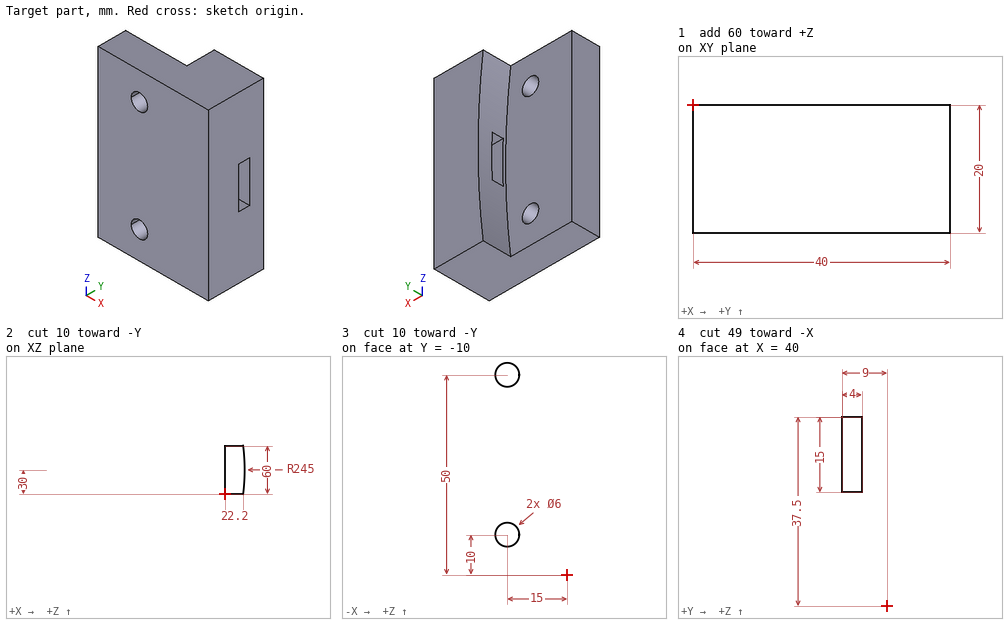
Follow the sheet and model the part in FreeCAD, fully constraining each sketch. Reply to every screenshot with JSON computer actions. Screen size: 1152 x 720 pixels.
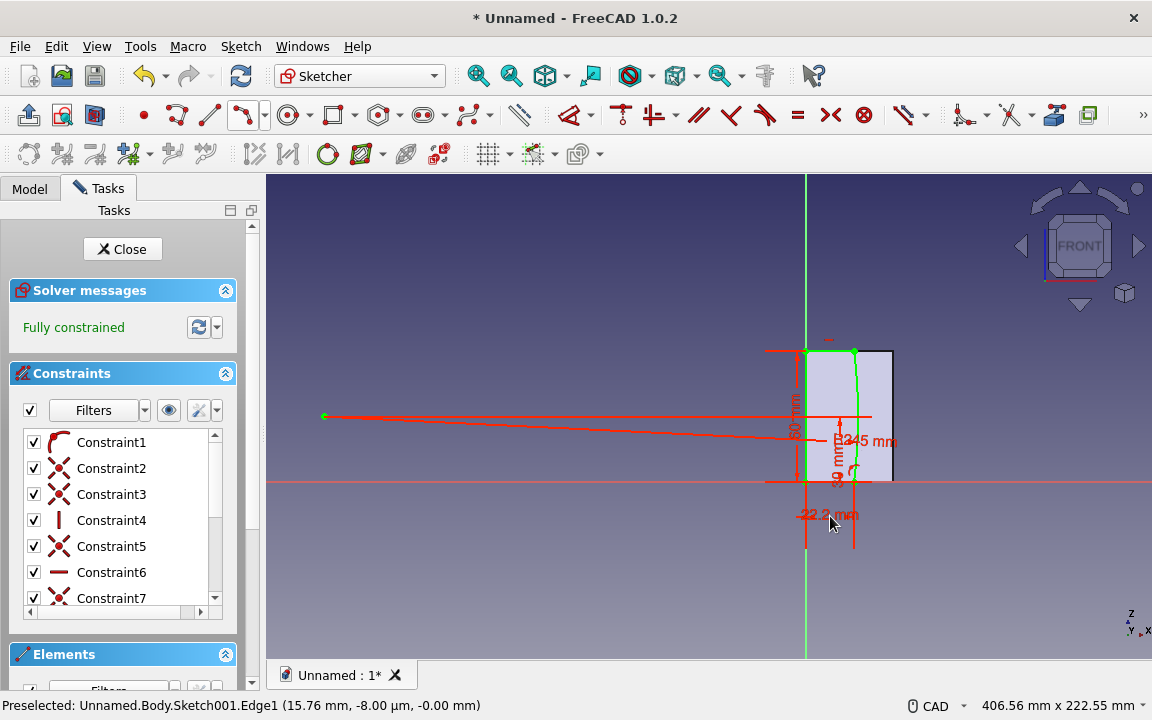
{"action": "left_click", "coordinate": [123, 249]}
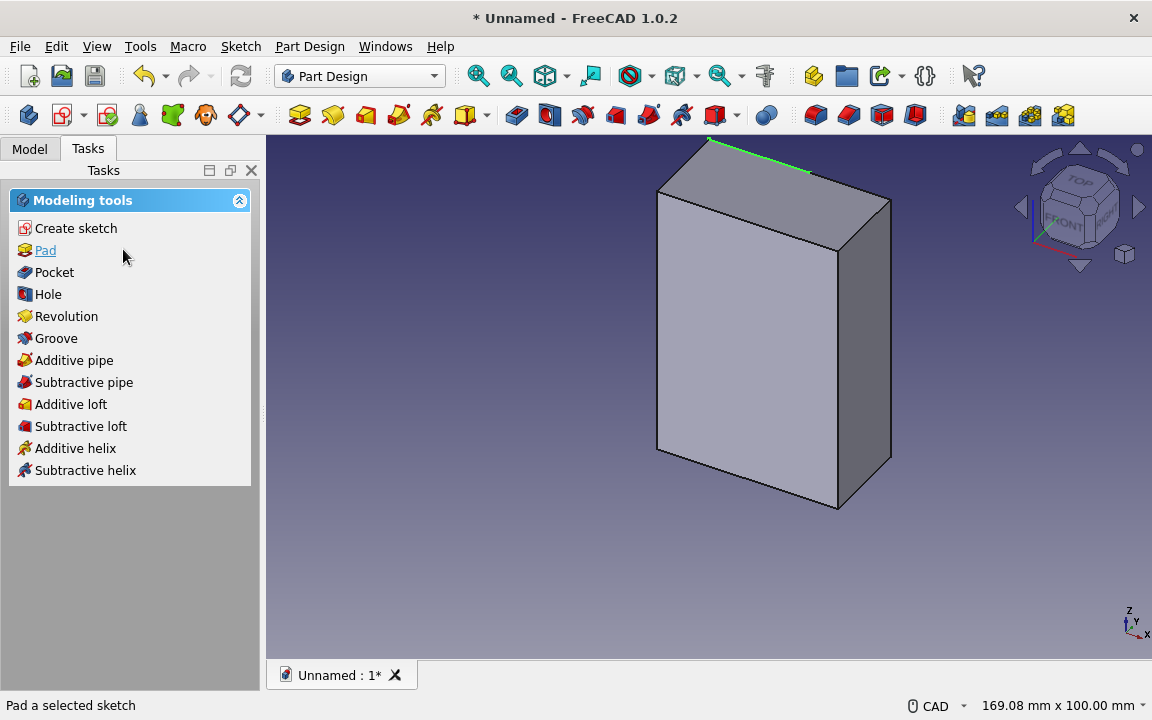
{"action": "left_click", "coordinate": [517, 116]}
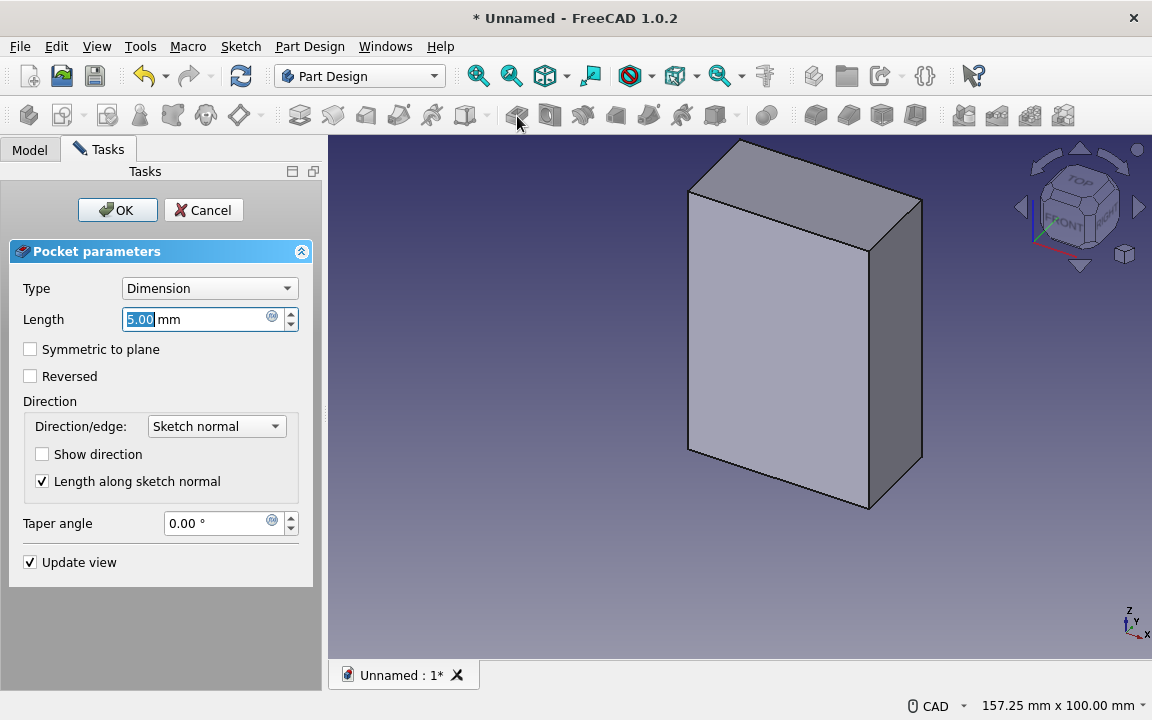
{"action": "type", "text": "10"}
{"action": "key", "text": "Tab"}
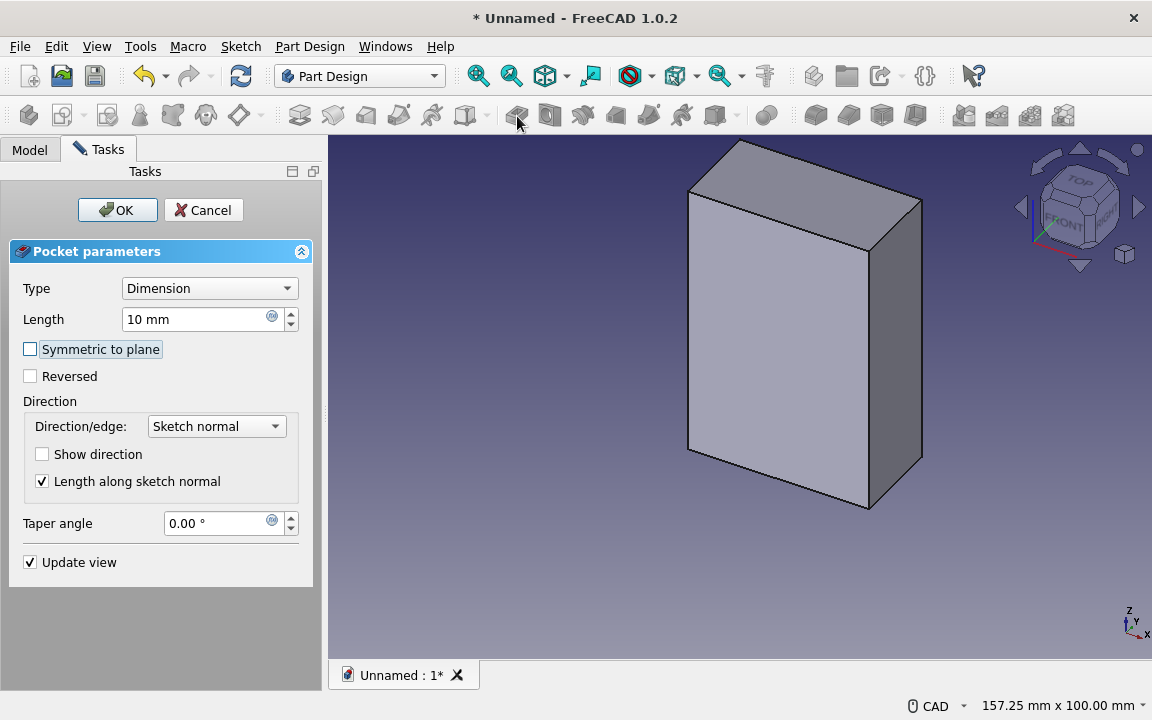
{"action": "left_click", "coordinate": [31, 376]}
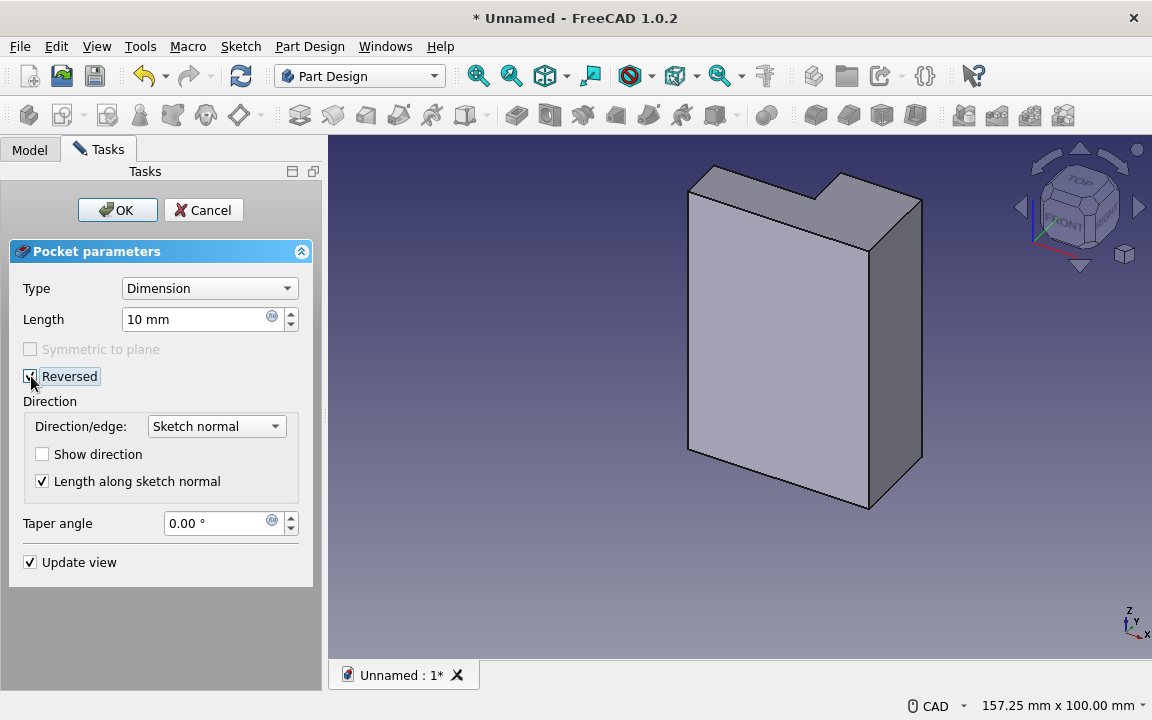
{"action": "left_click", "coordinate": [118, 210]}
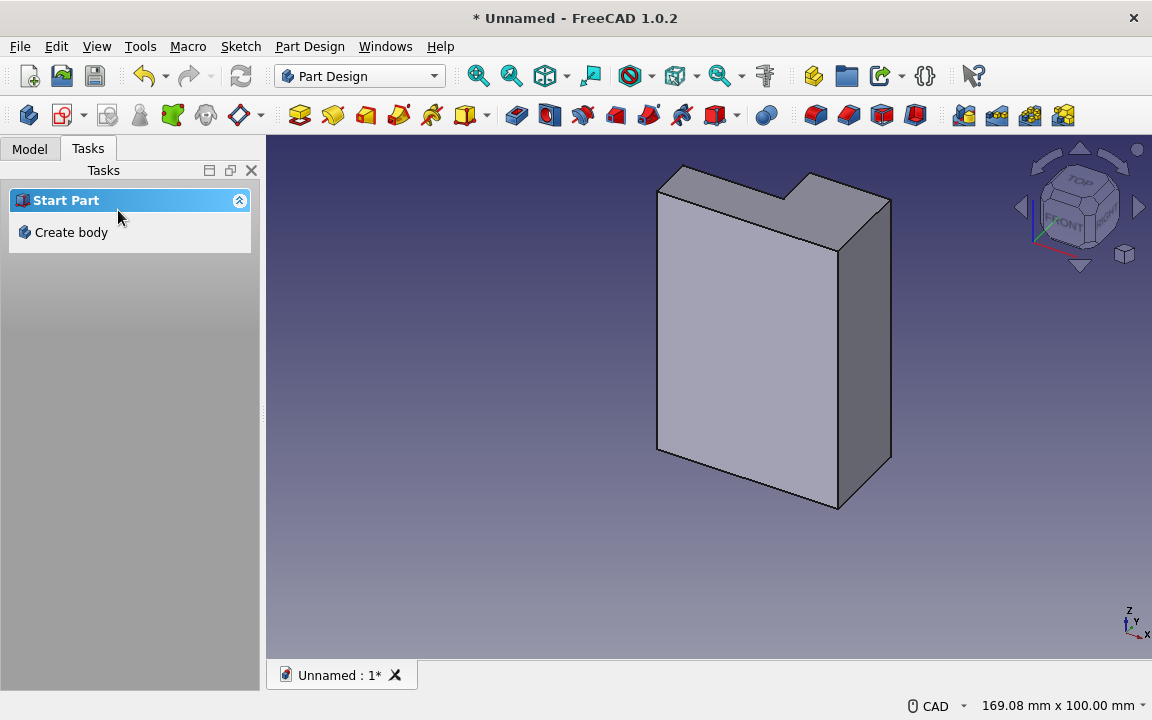
{"action": "key", "text": "4"}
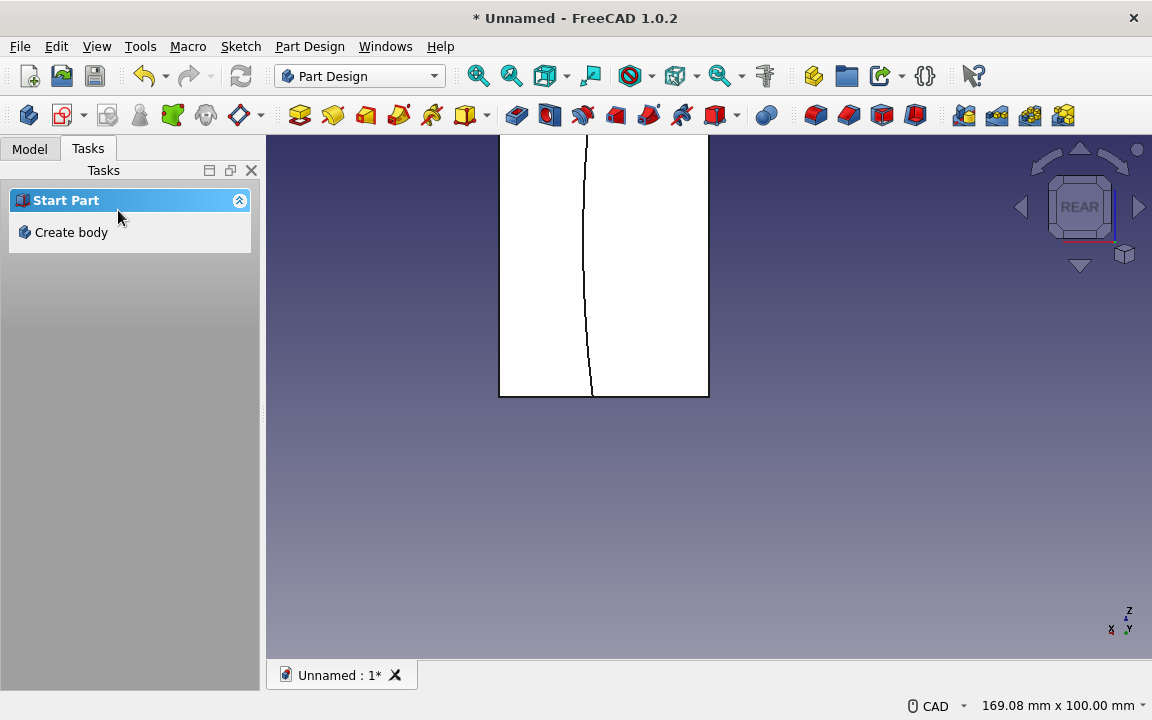
{"action": "left_click", "coordinate": [479, 76]}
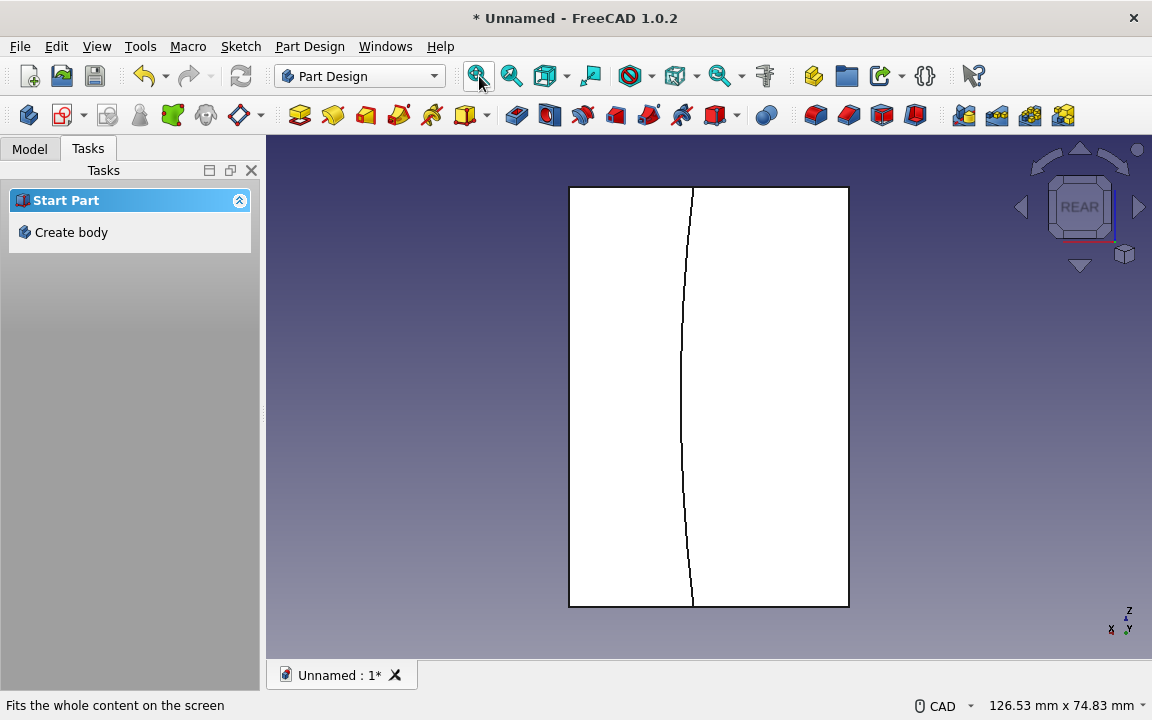
{"action": "left_click", "coordinate": [765, 396]}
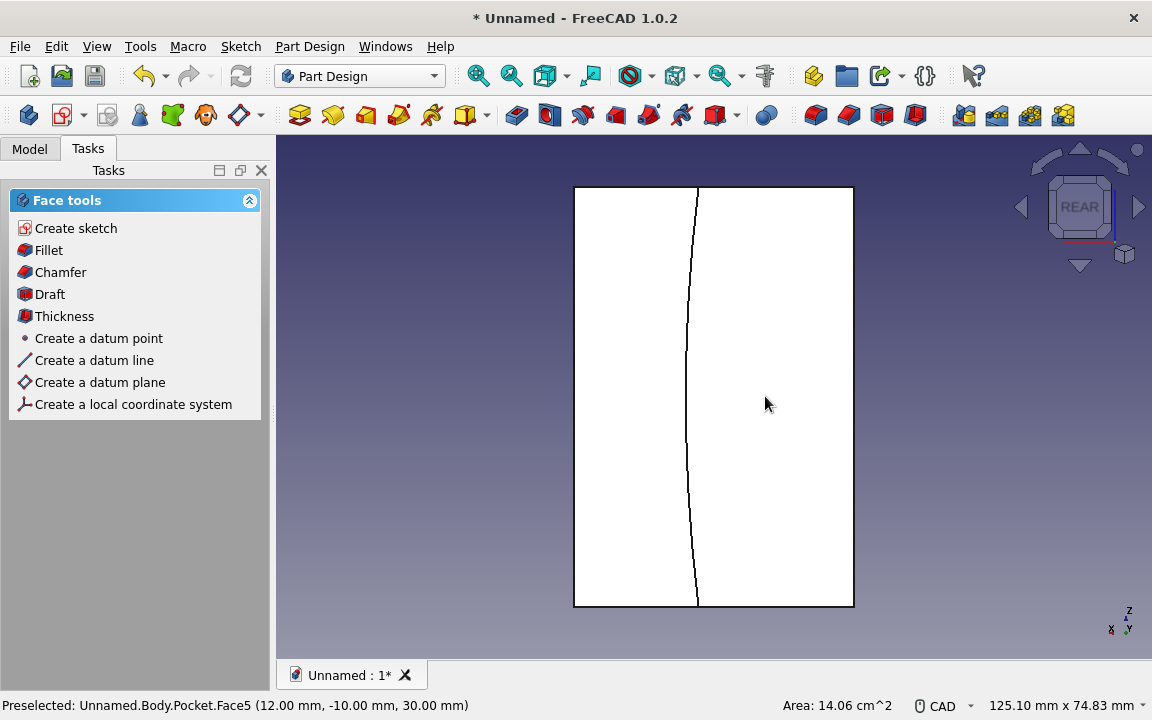
{"action": "left_click", "coordinate": [62, 116]}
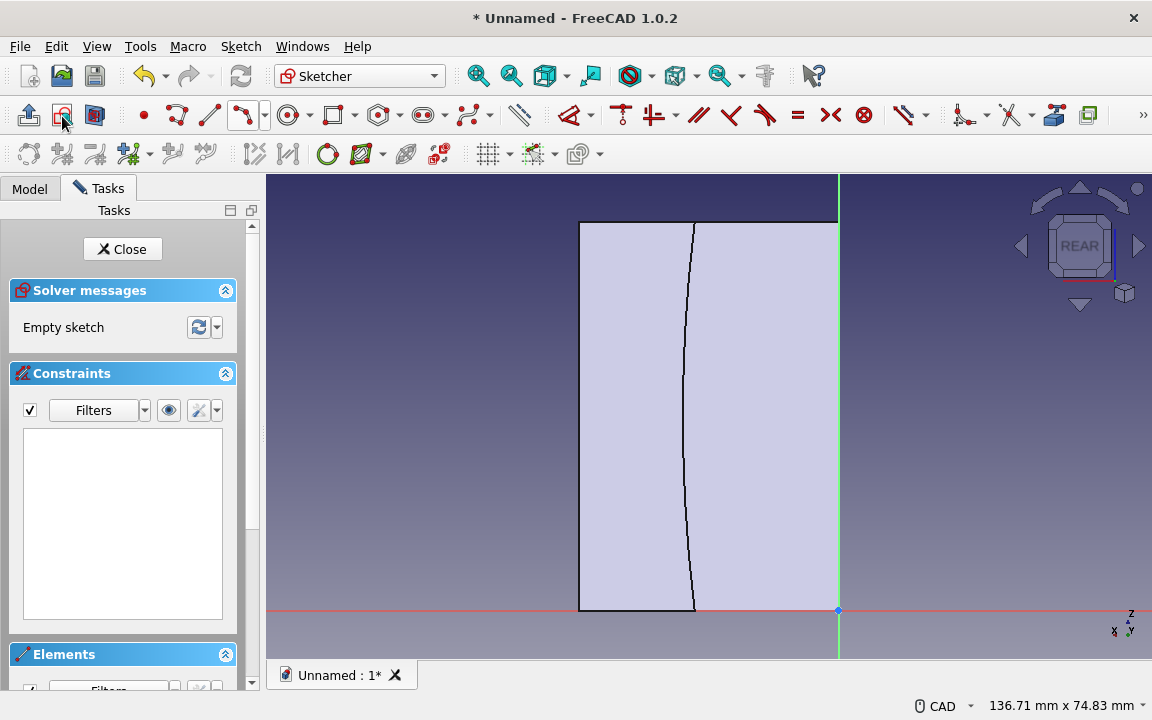
{"action": "scroll", "coordinate": [294, 314], "scroll_direction": "down", "scroll_amount": 1}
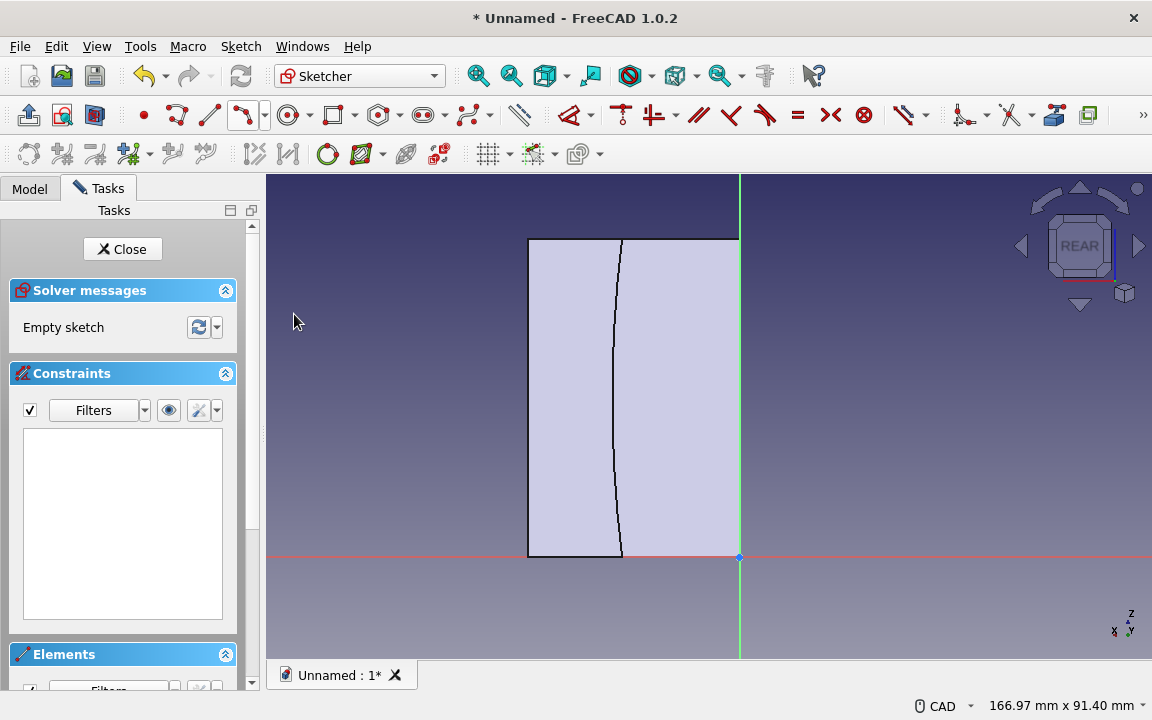
{"action": "left_click", "coordinate": [288, 116]}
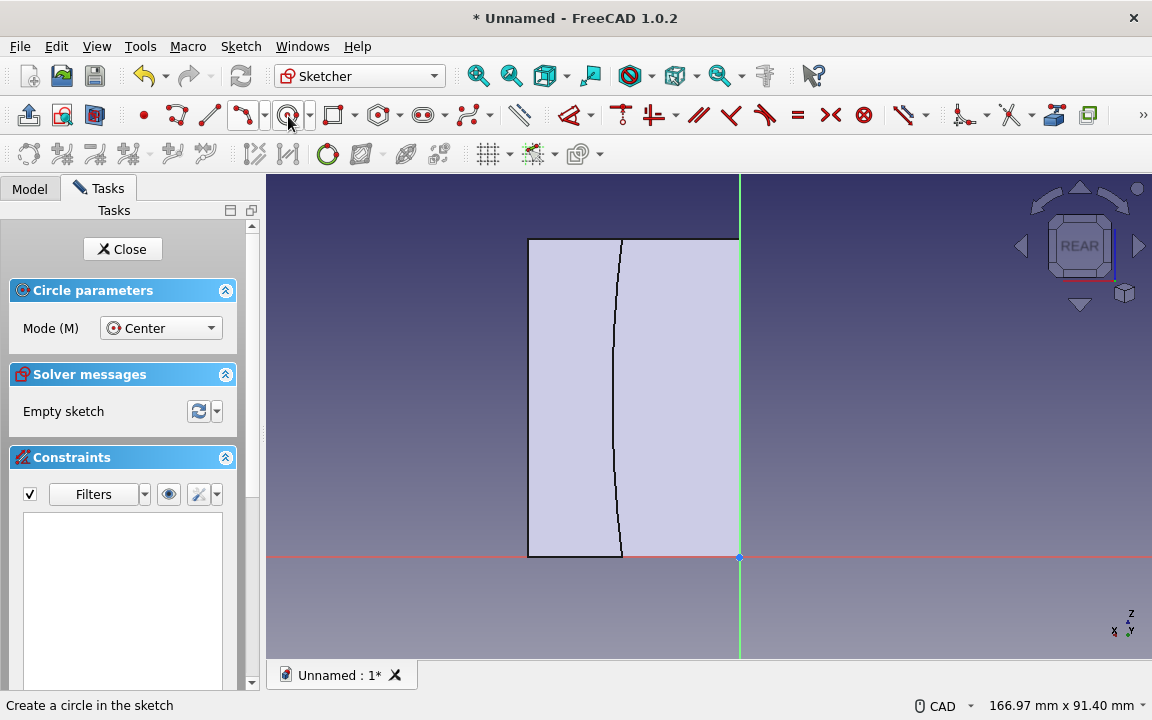
{"action": "scroll", "coordinate": [660, 504], "scroll_direction": "up", "scroll_amount": 2}